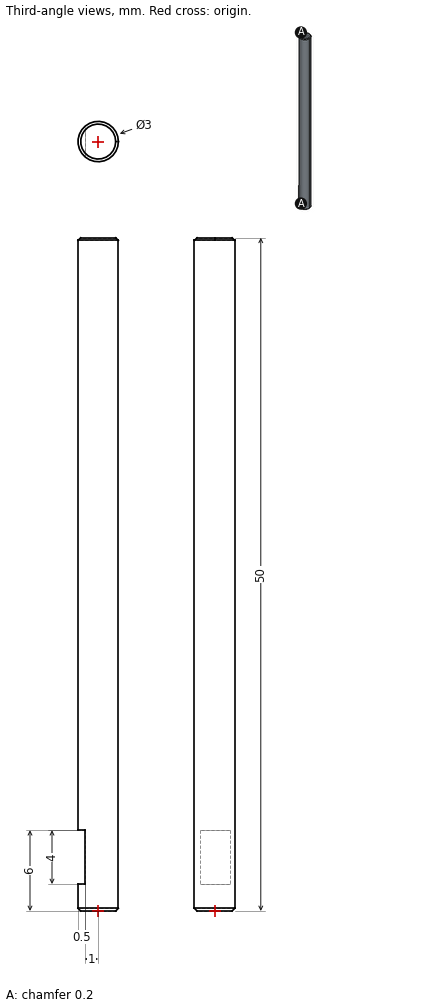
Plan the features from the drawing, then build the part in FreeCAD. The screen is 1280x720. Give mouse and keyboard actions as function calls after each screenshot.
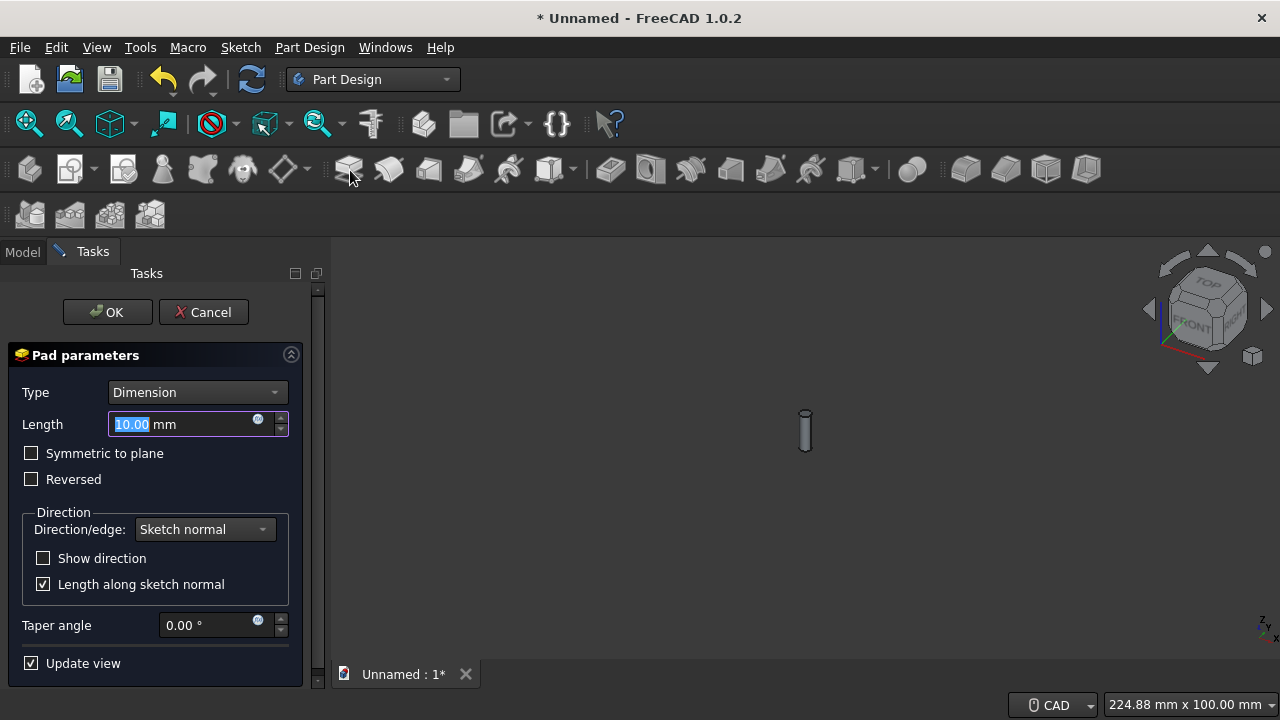
text(50)
key(Tab)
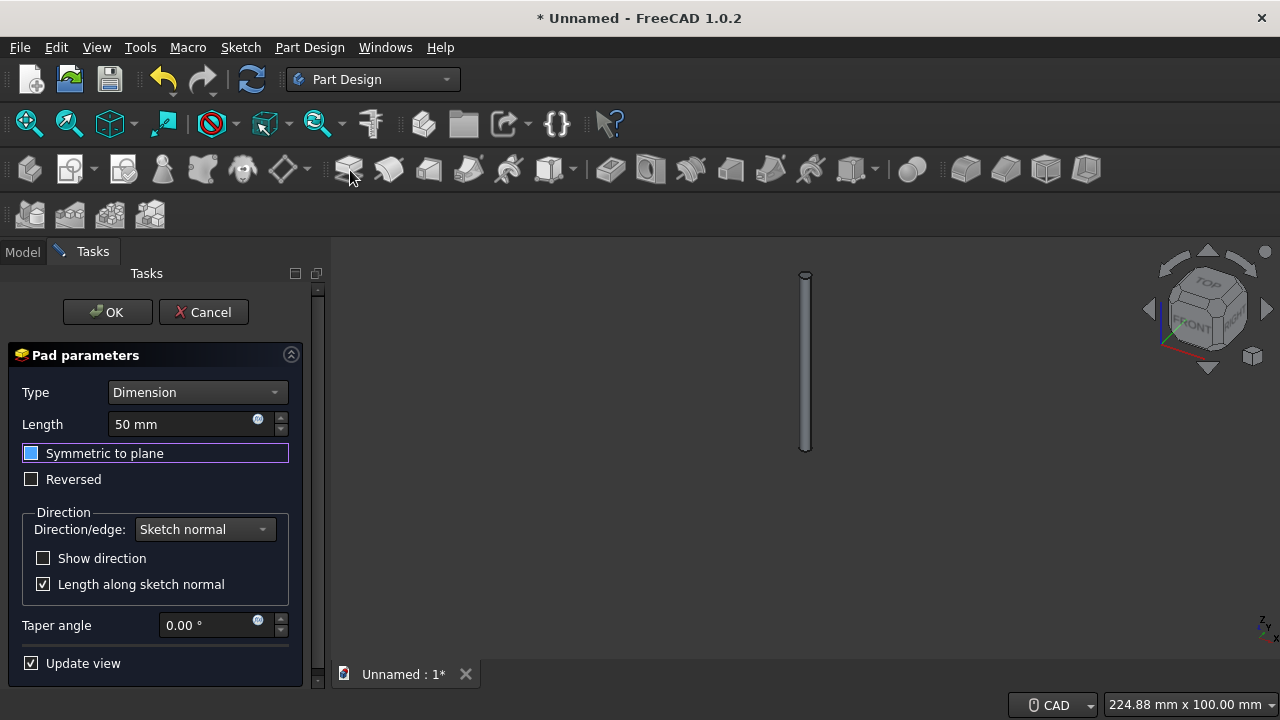
click(108, 312)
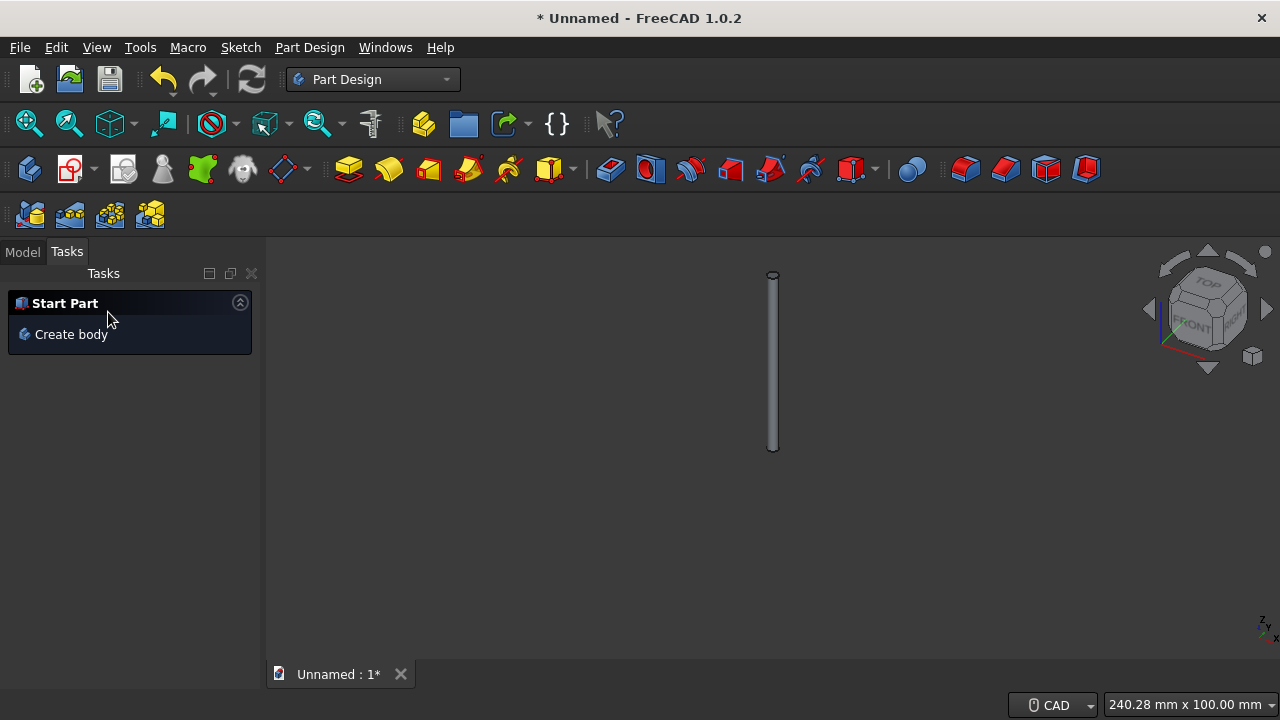
click(30, 124)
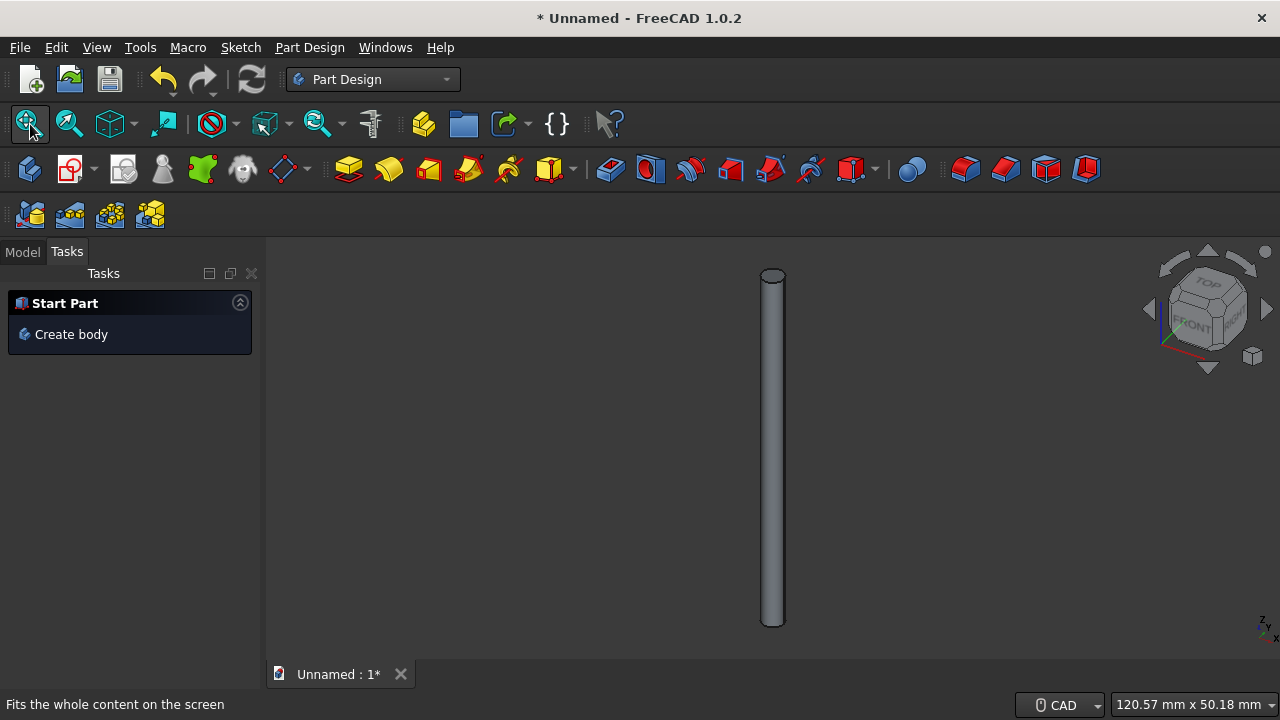
click(70, 170)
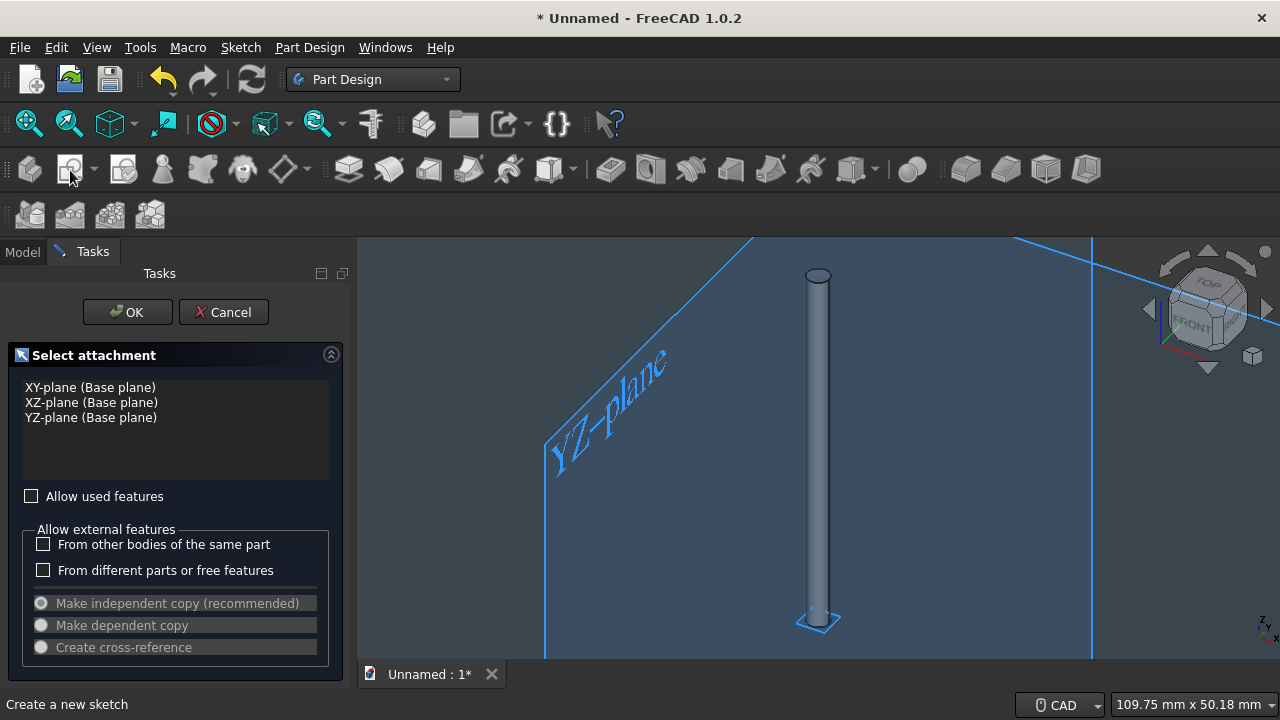
click(82, 402)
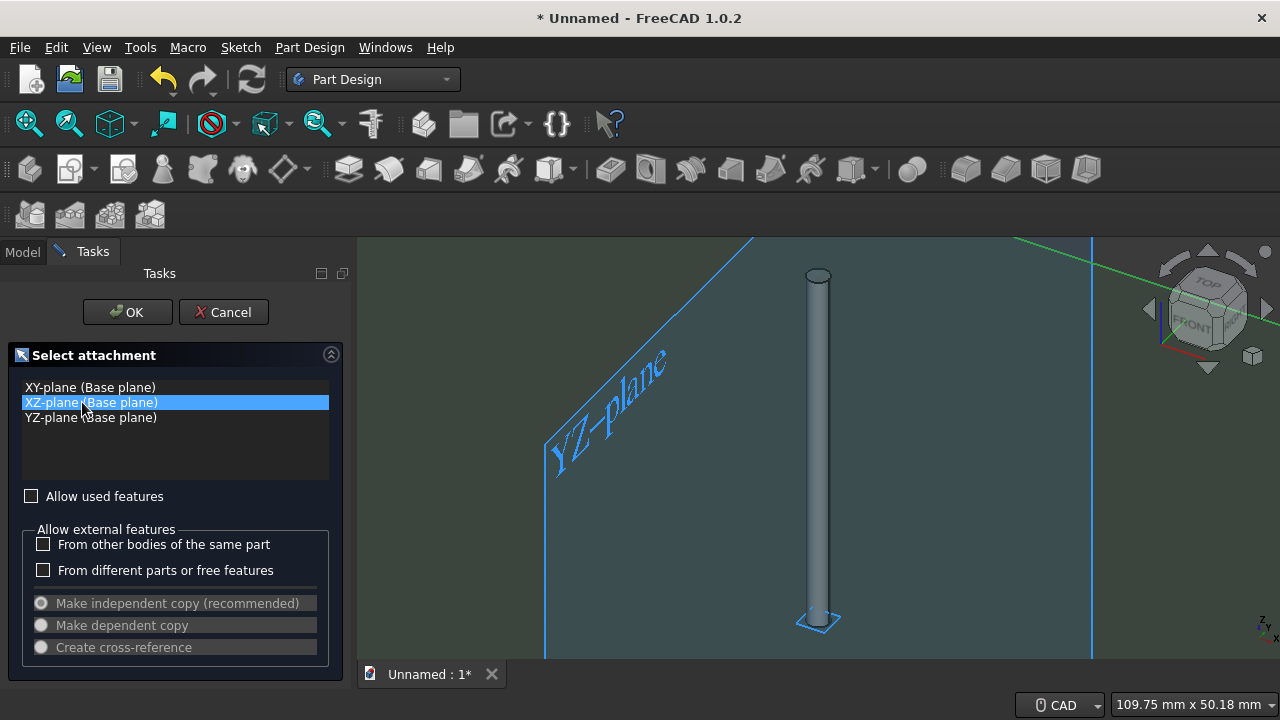
click(128, 312)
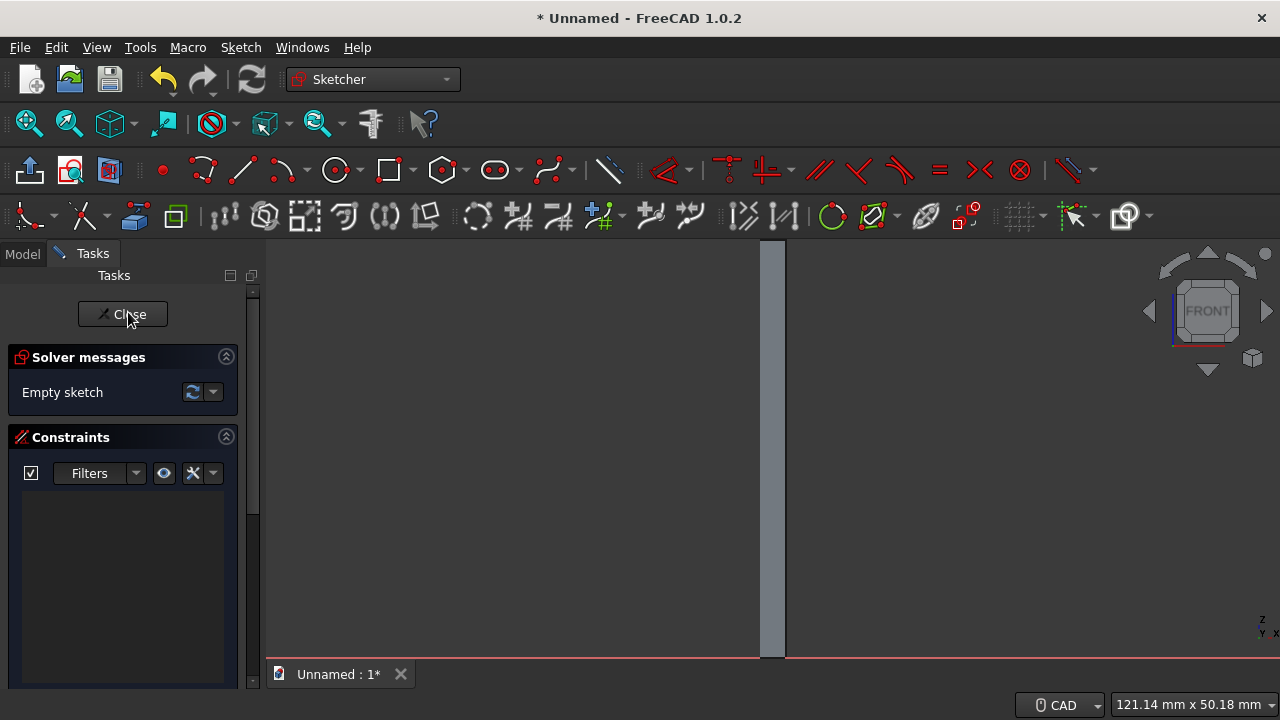
click(110, 170)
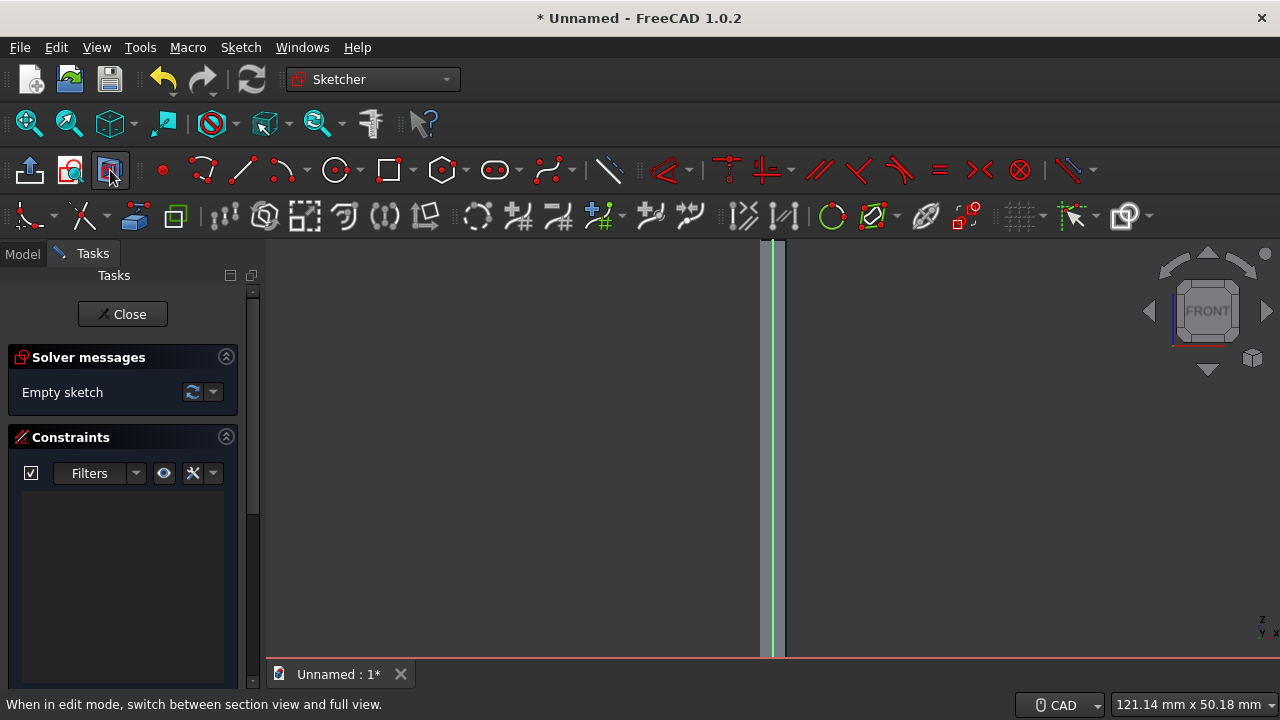
scroll(704, 449, down, 5)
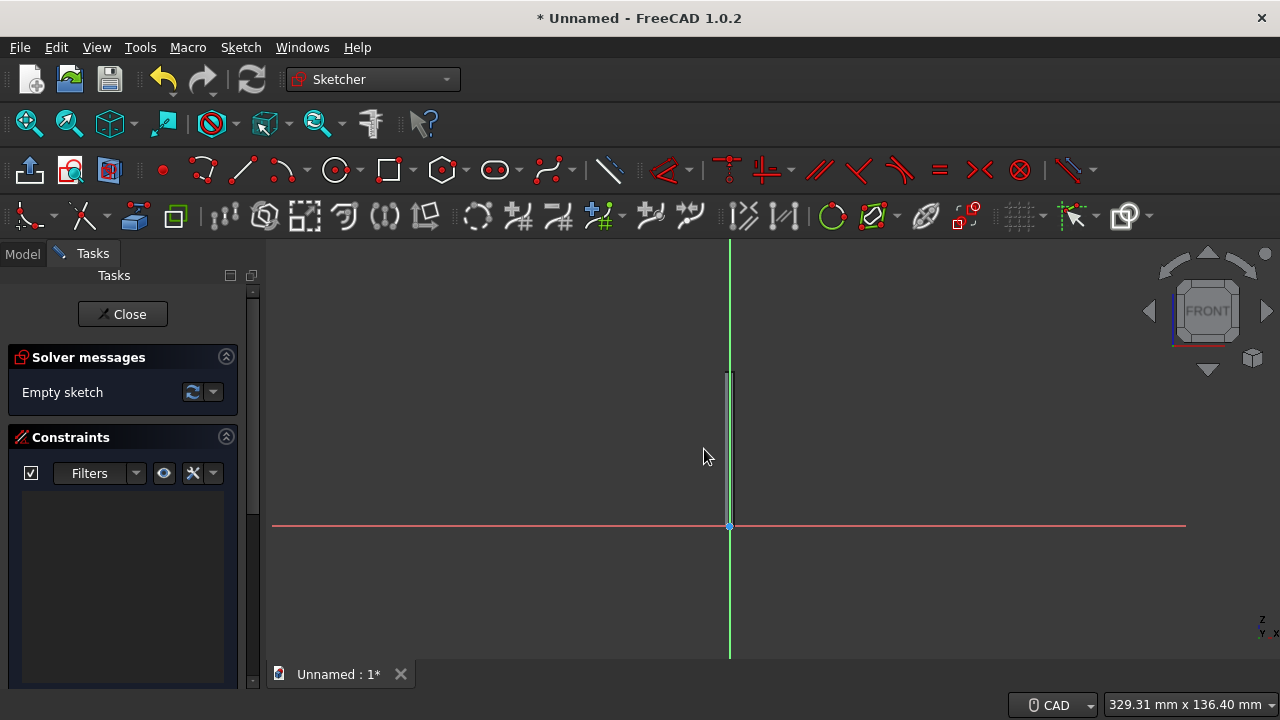
scroll(729, 523, up, 13)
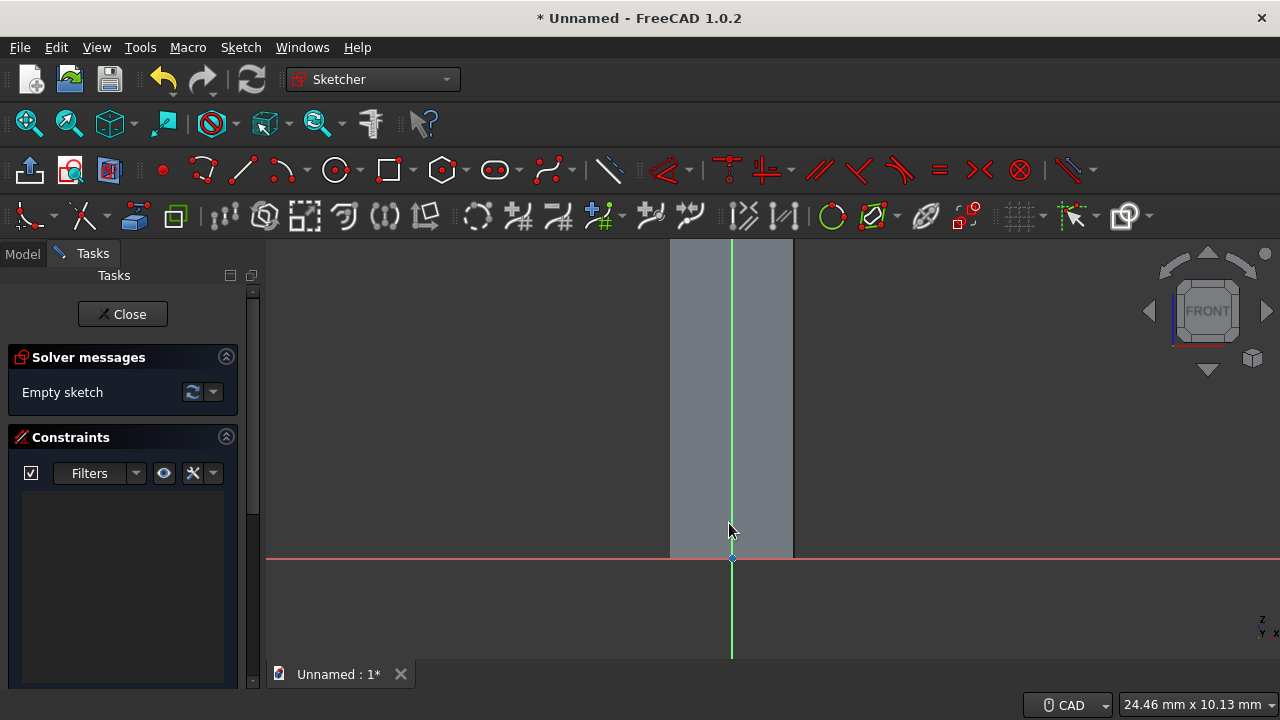
click(390, 170)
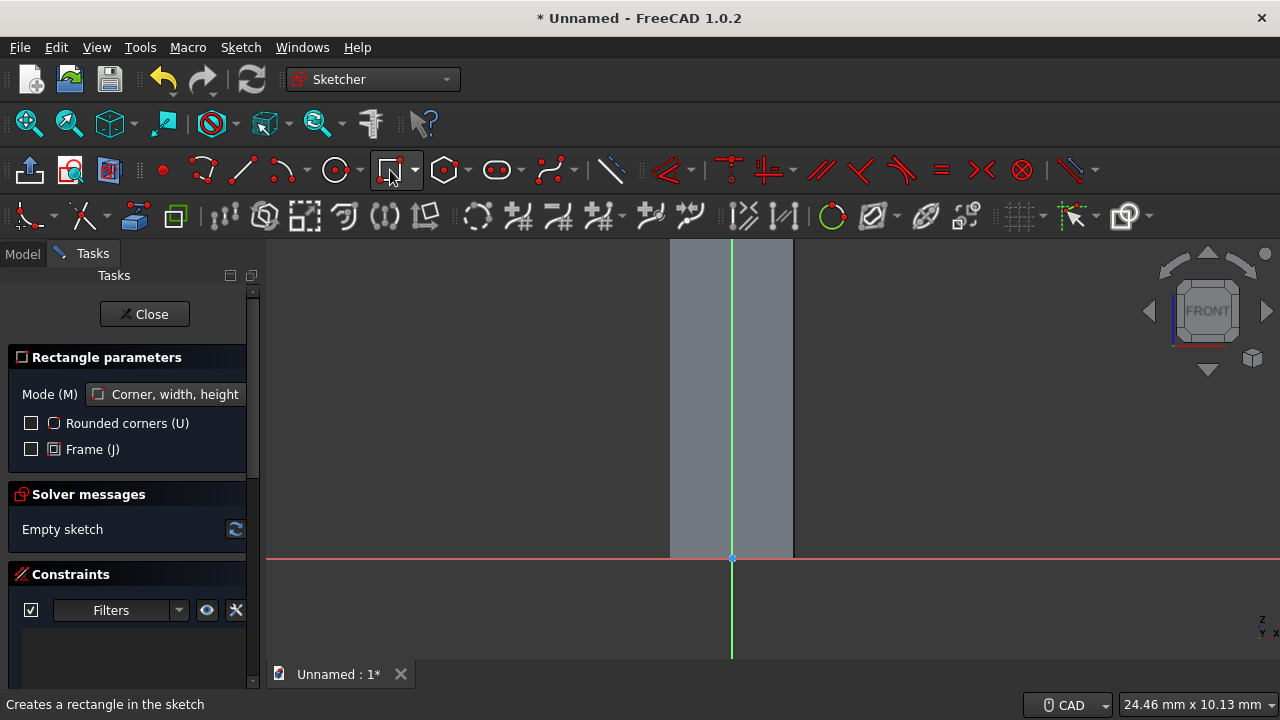
click(670, 310)
click(691, 476)
key(Escape)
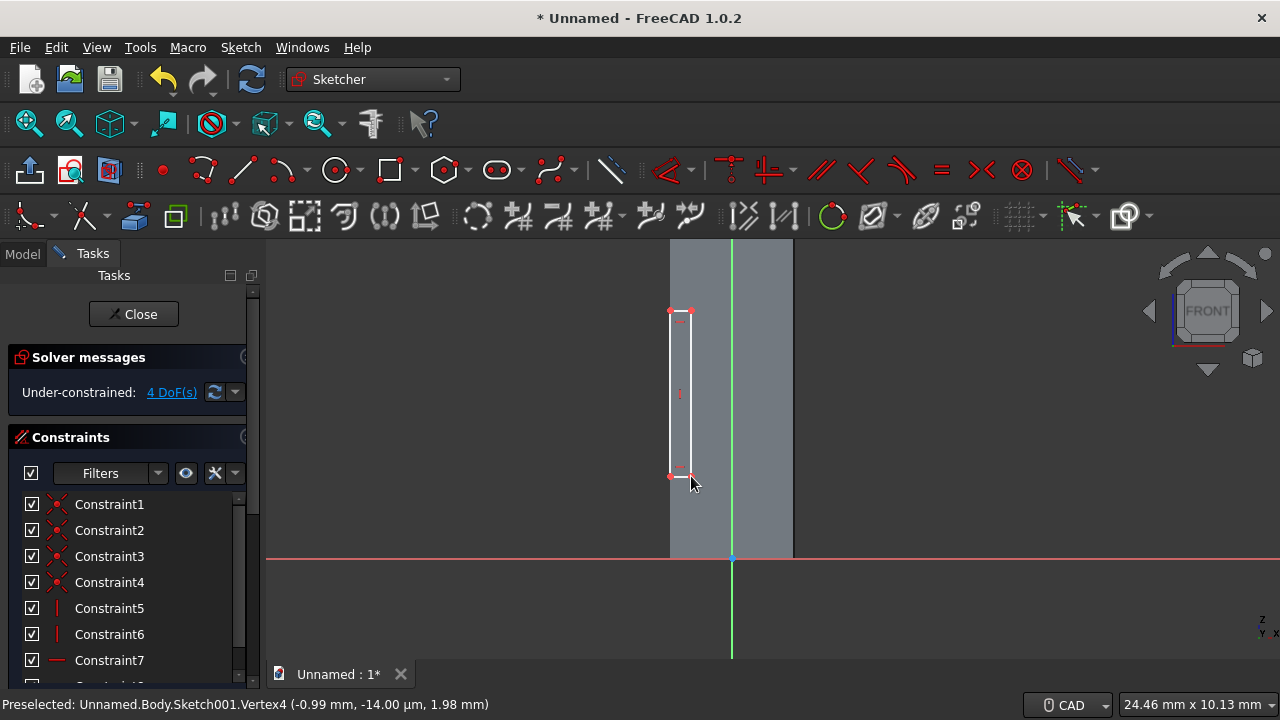
click(666, 170)